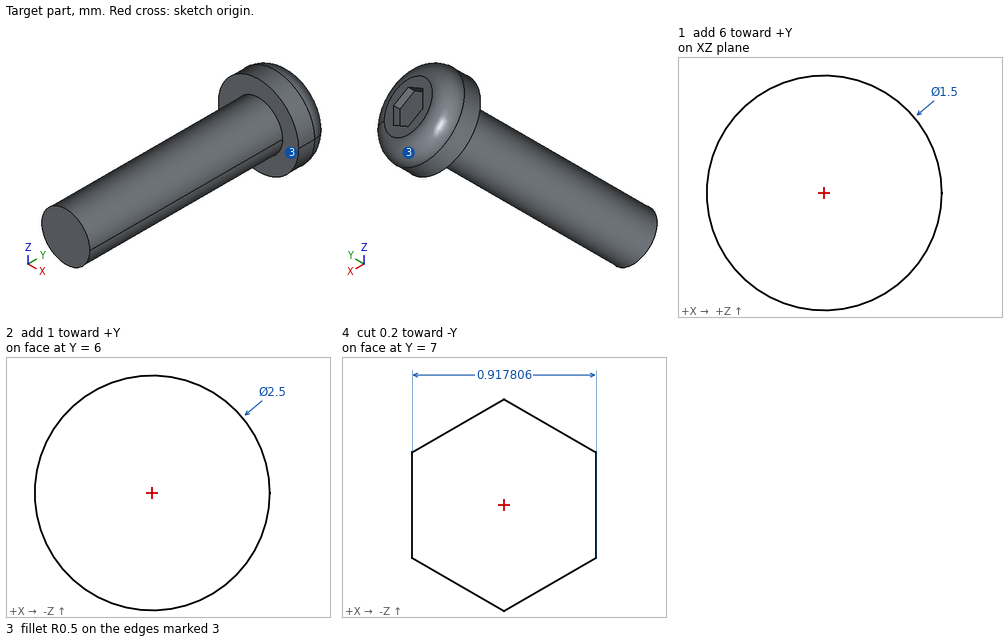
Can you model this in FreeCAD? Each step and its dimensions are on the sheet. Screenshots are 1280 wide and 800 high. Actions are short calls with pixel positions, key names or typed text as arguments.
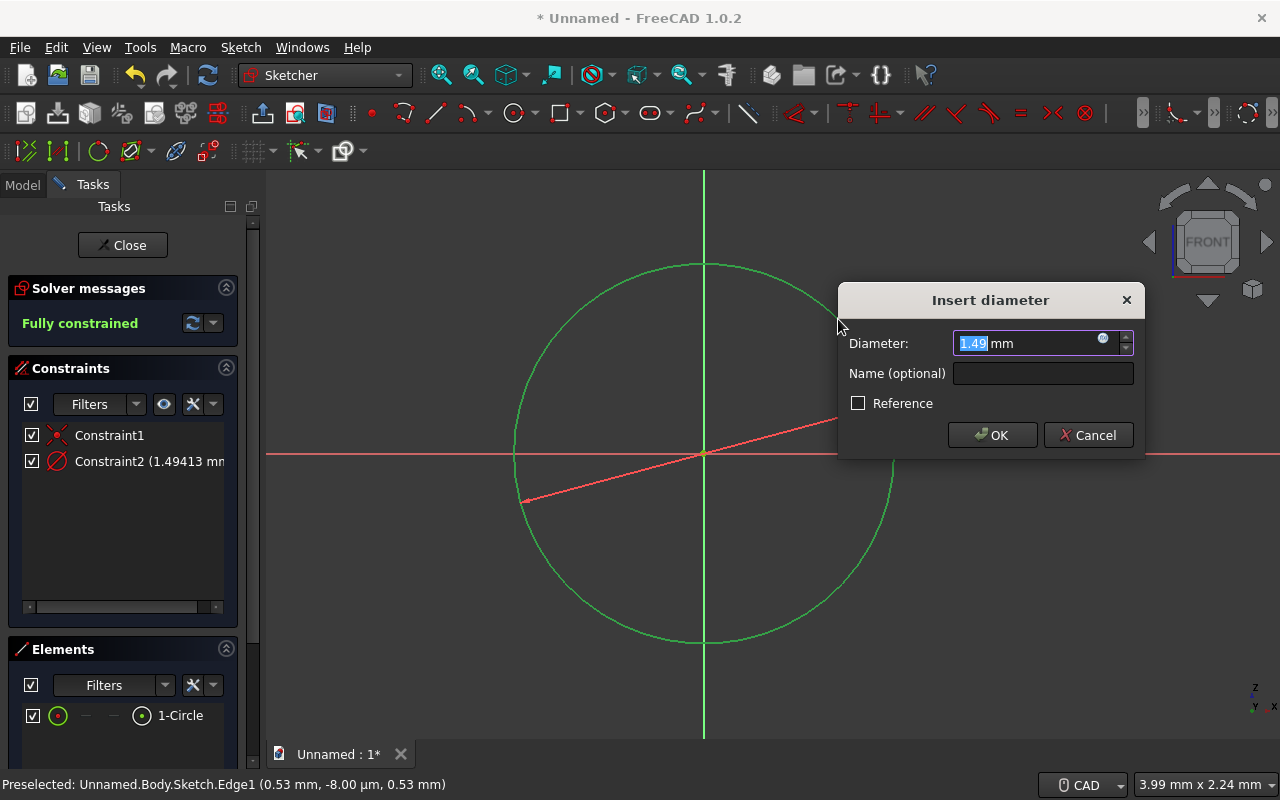
text(1.5)
key(Return)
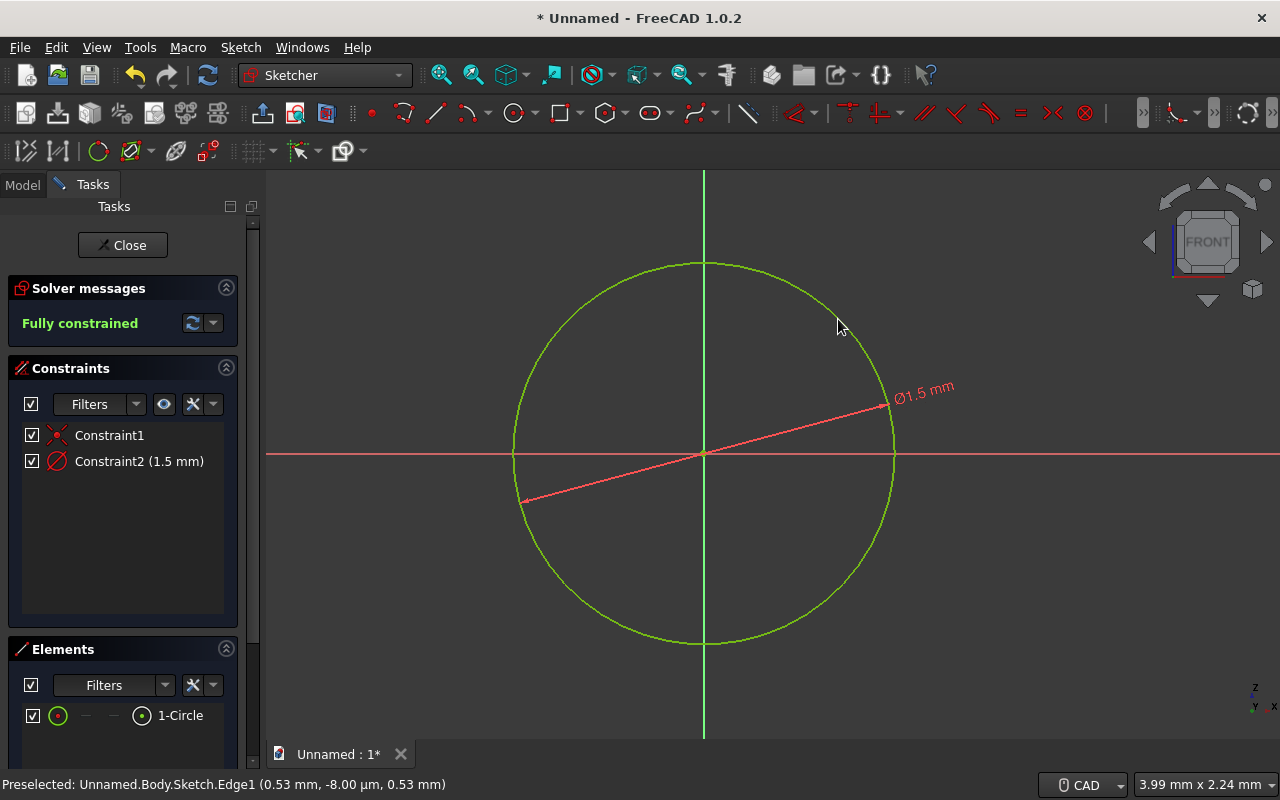
click(123, 245)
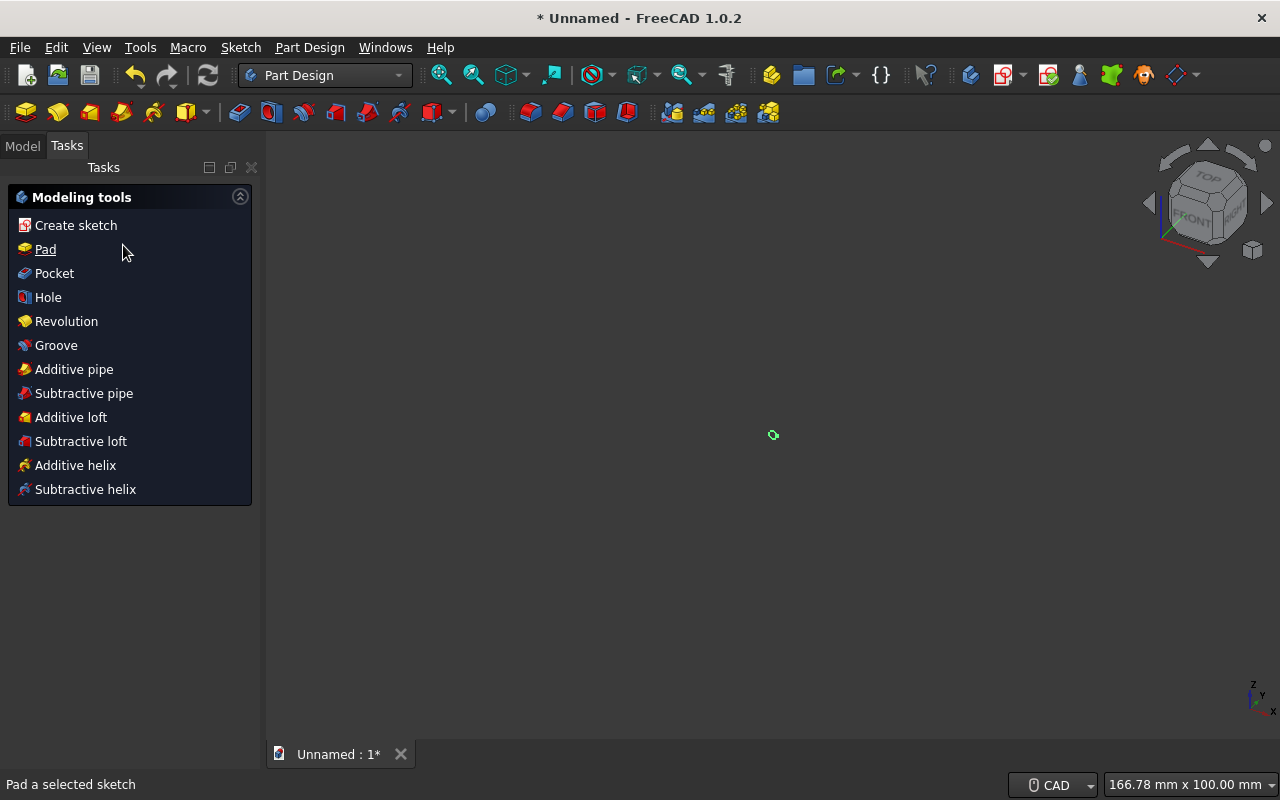
click(26, 112)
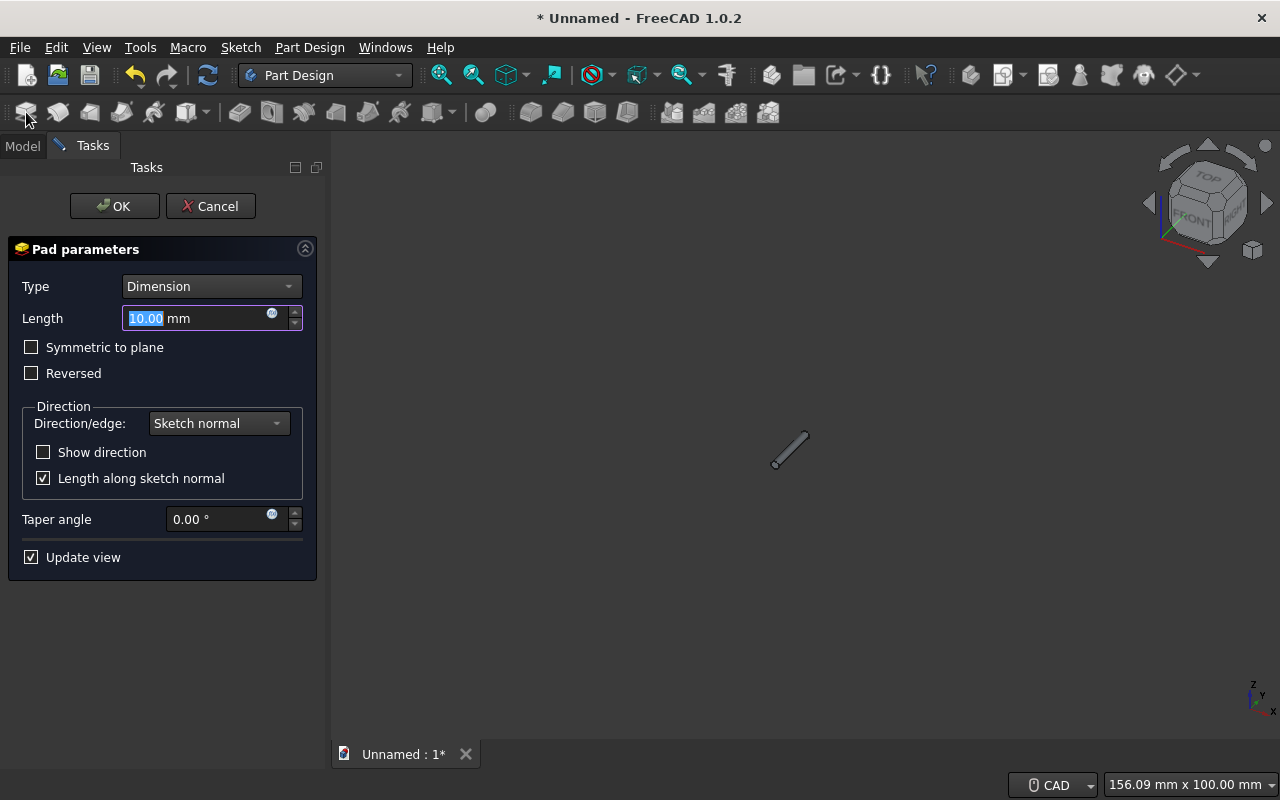
text(6)
key(Tab)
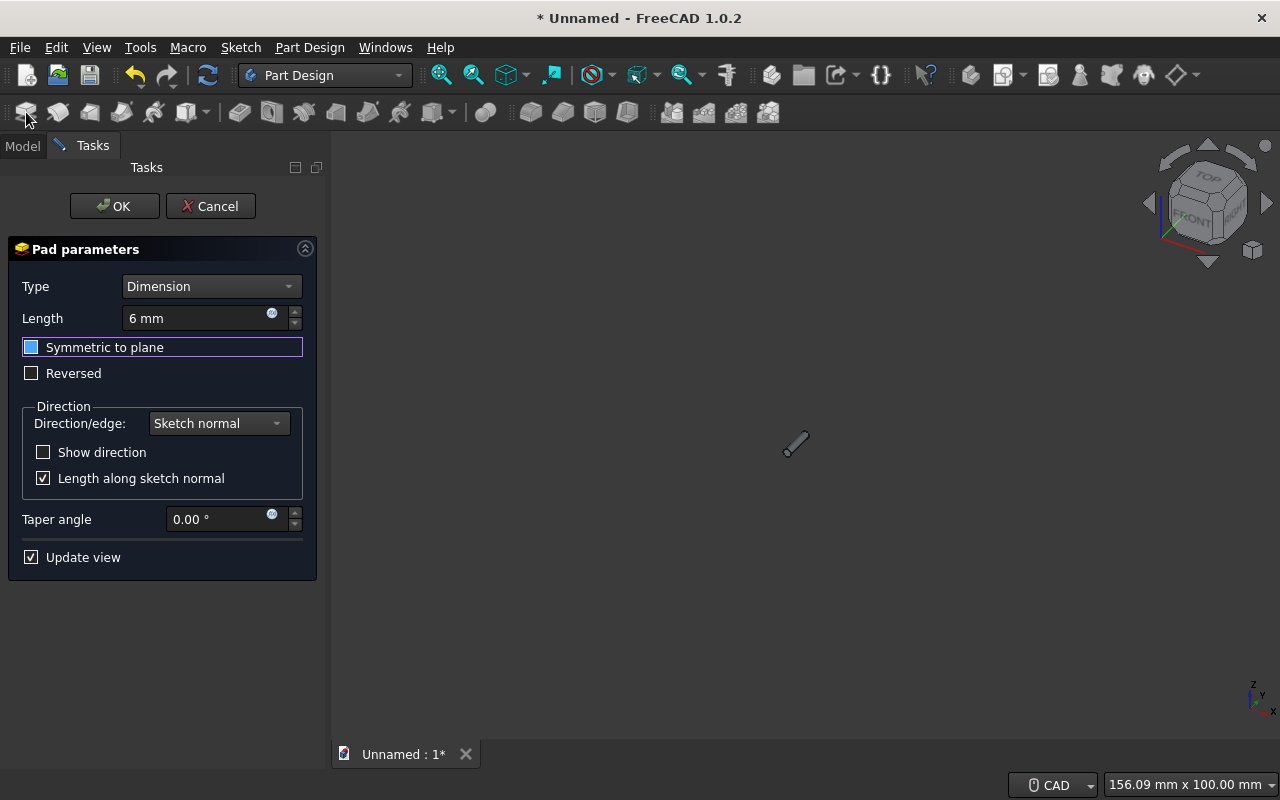
click(30, 373)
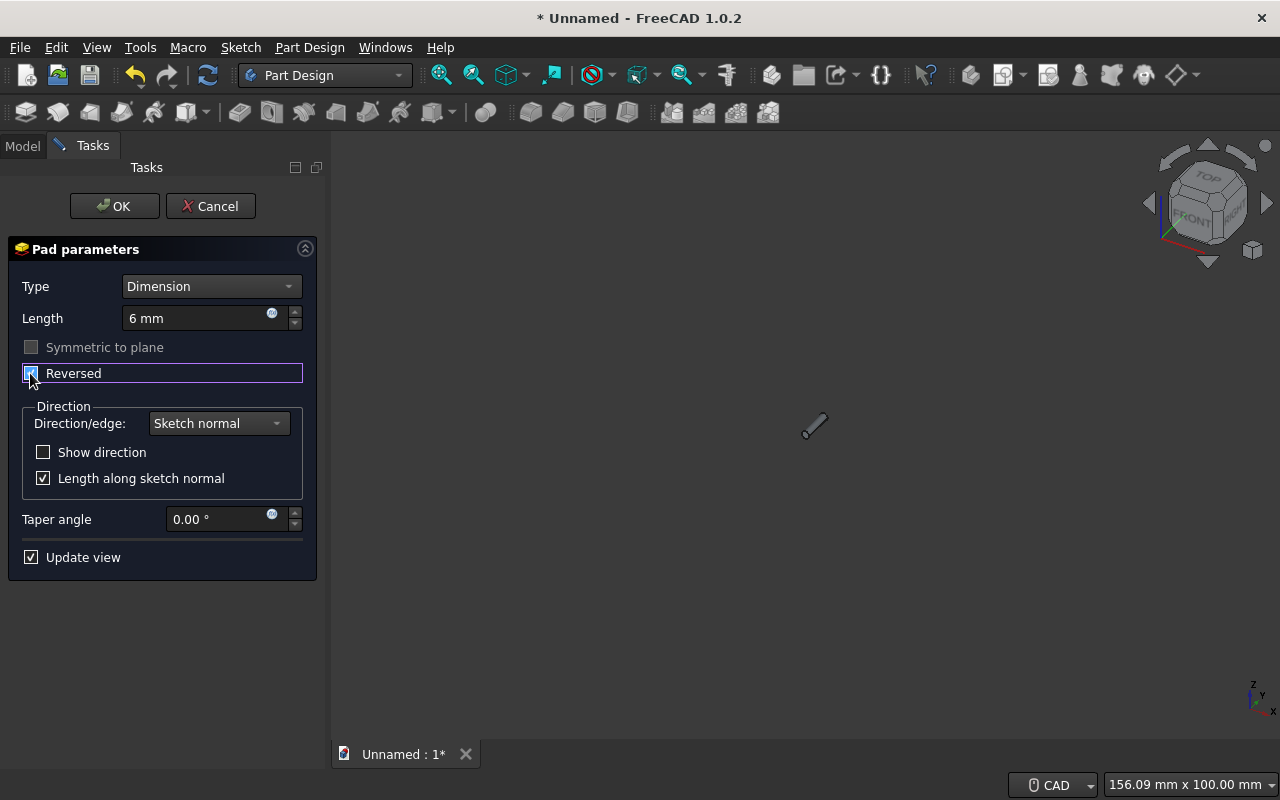
click(115, 206)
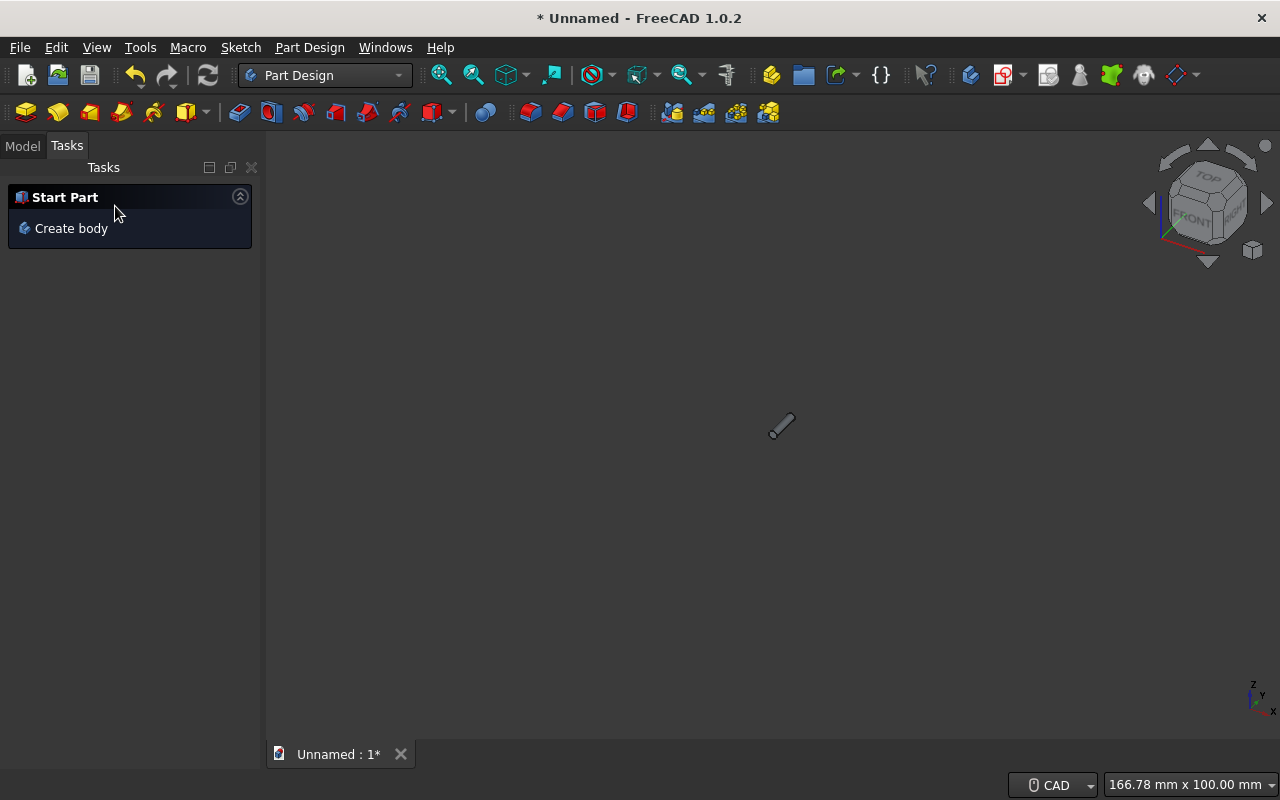
click(442, 76)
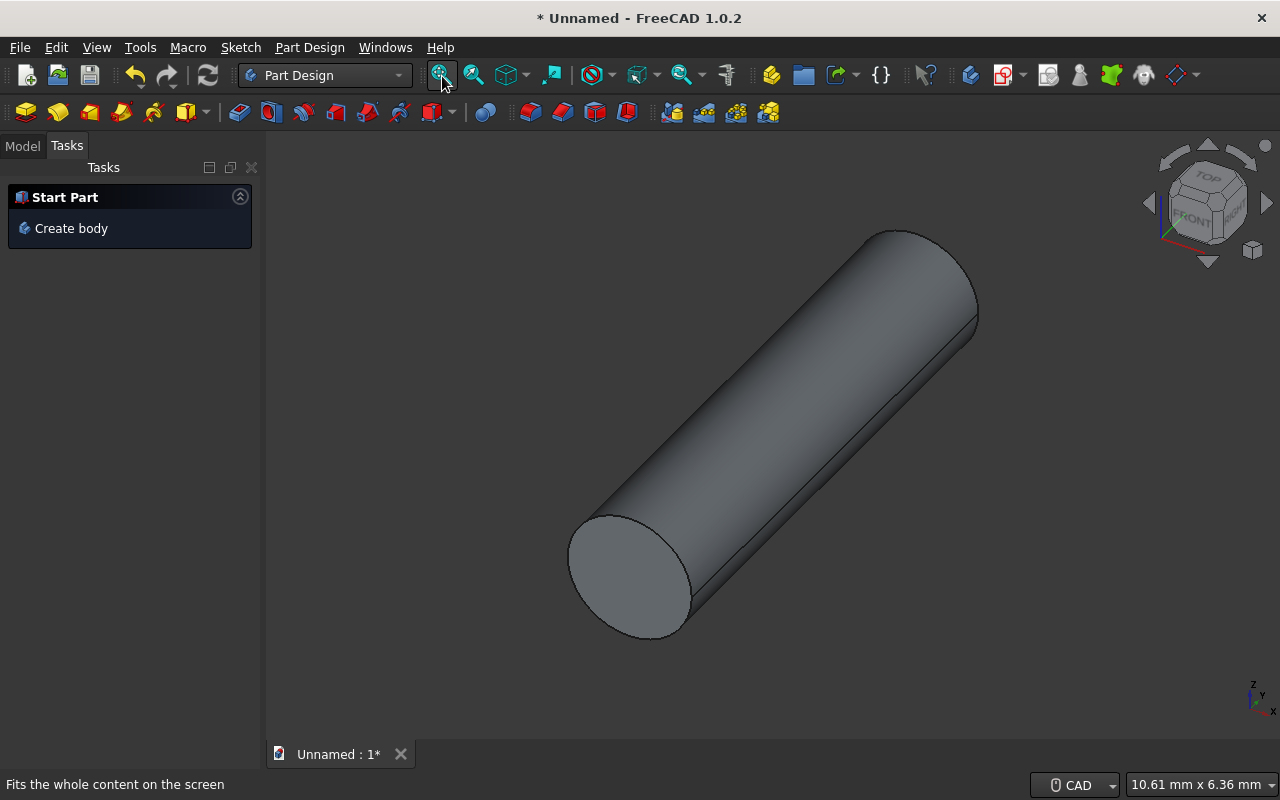
key(4)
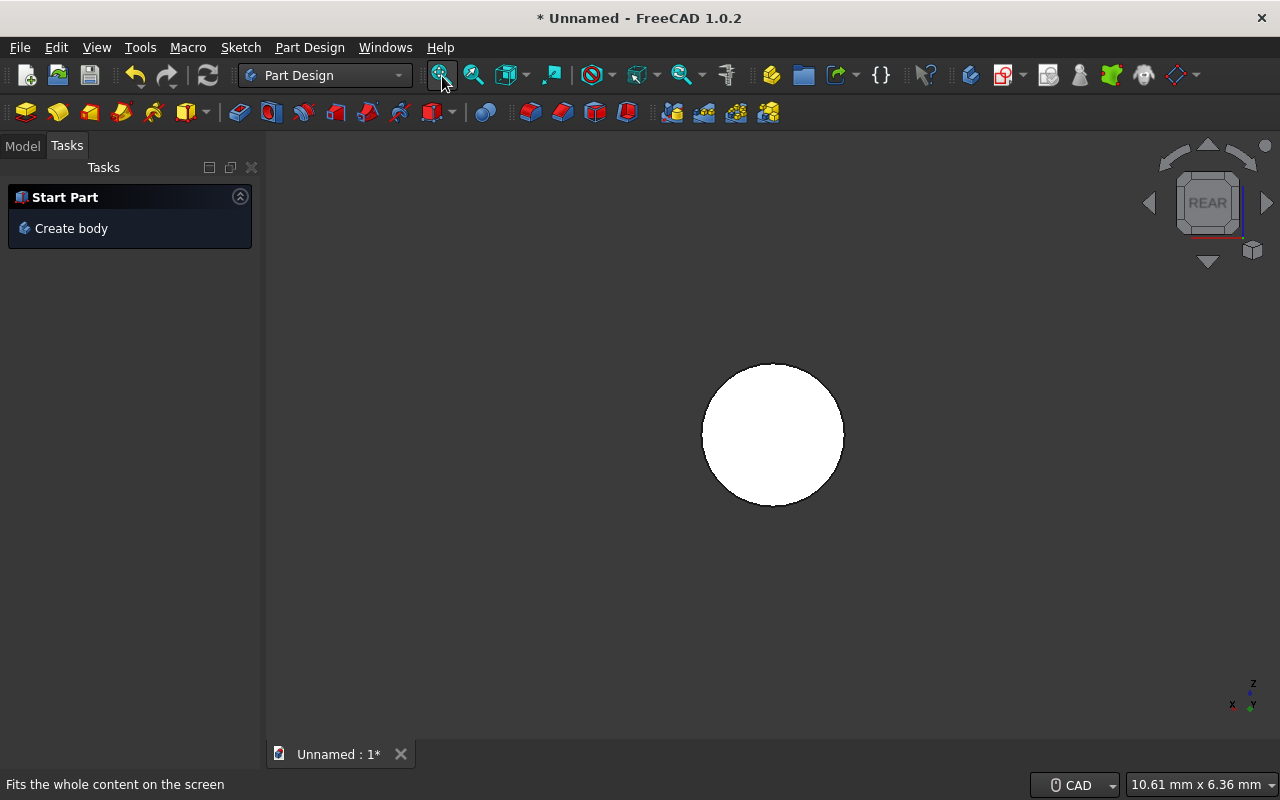
click(442, 76)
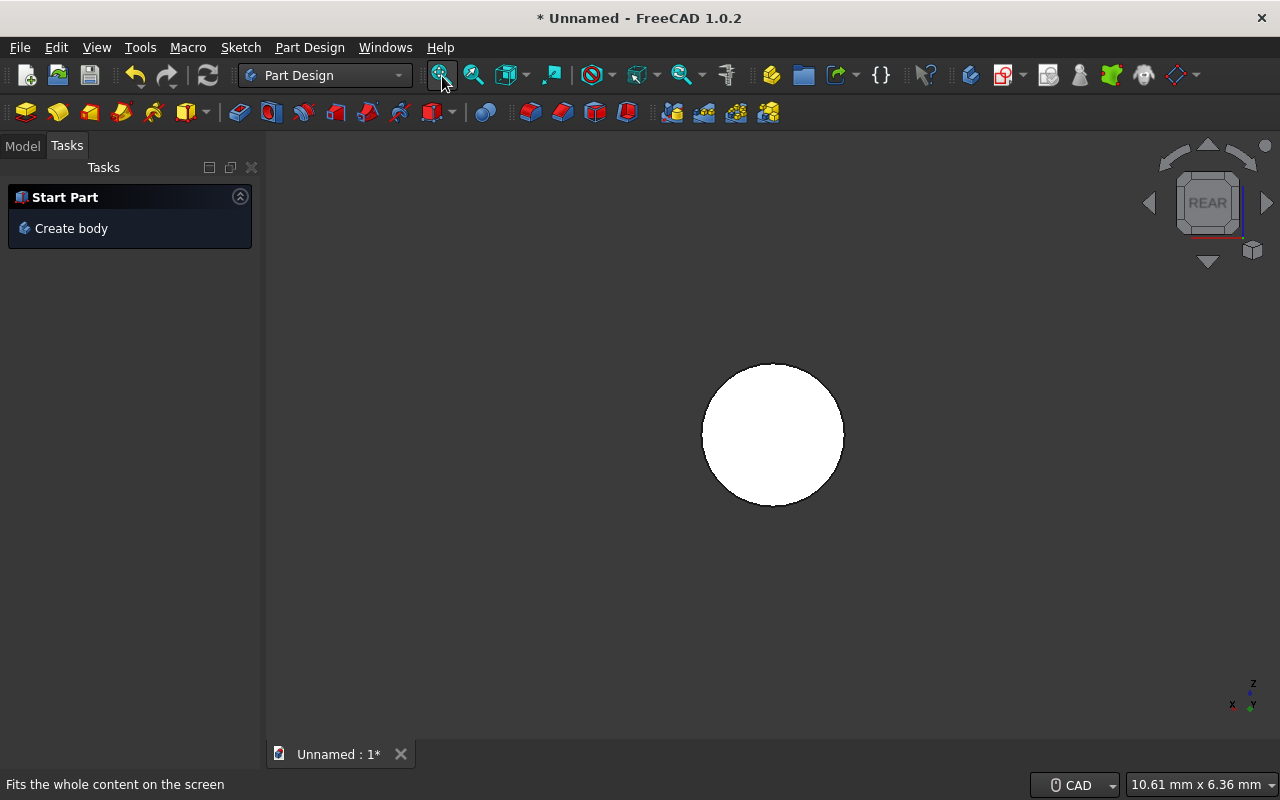
click(773, 434)